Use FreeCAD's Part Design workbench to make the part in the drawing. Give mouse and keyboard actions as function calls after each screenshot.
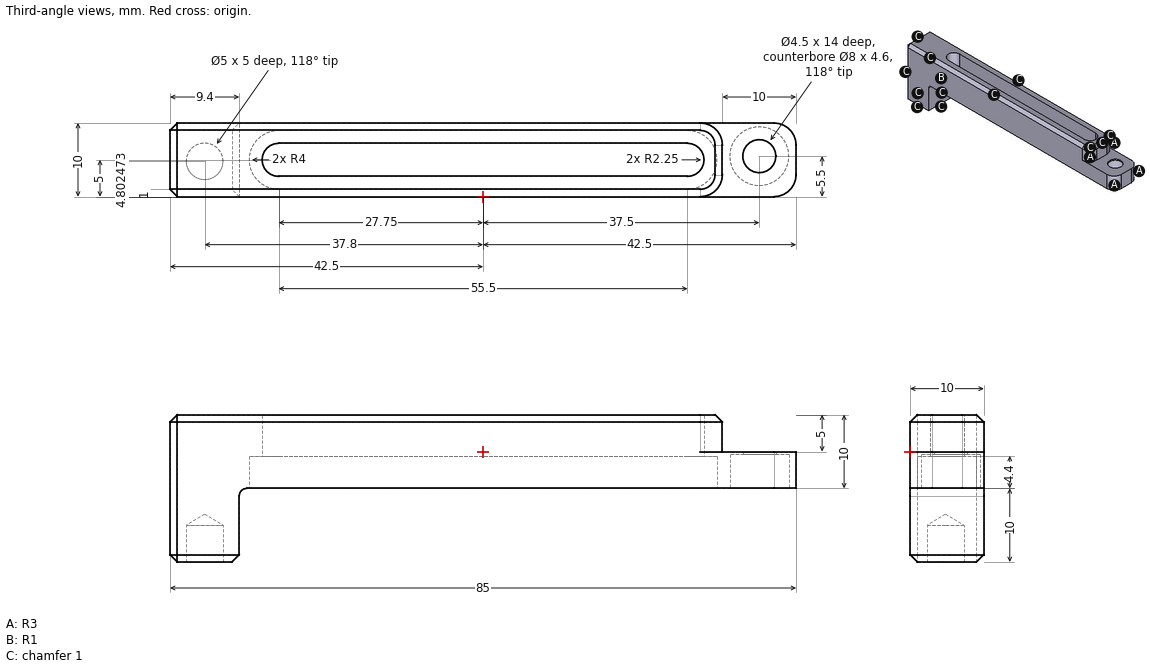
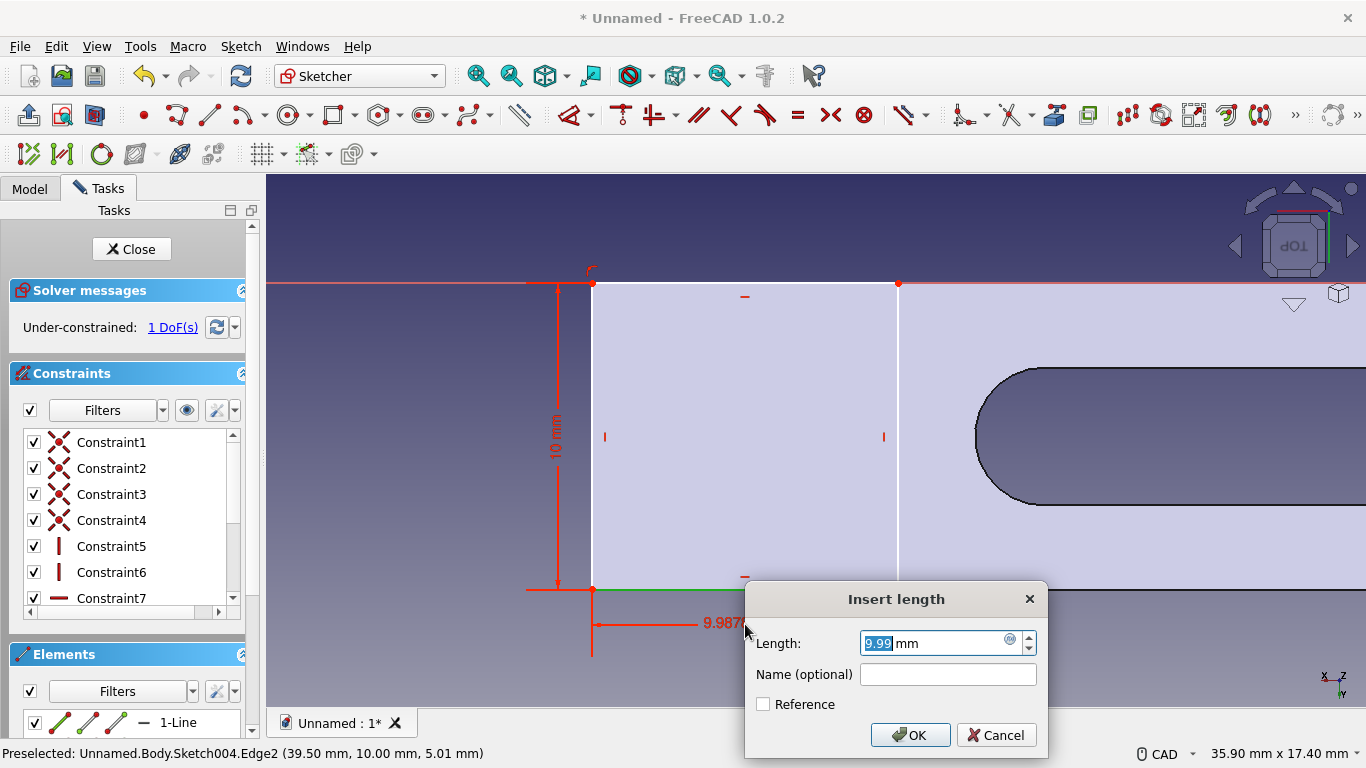
text(10)
key(Return)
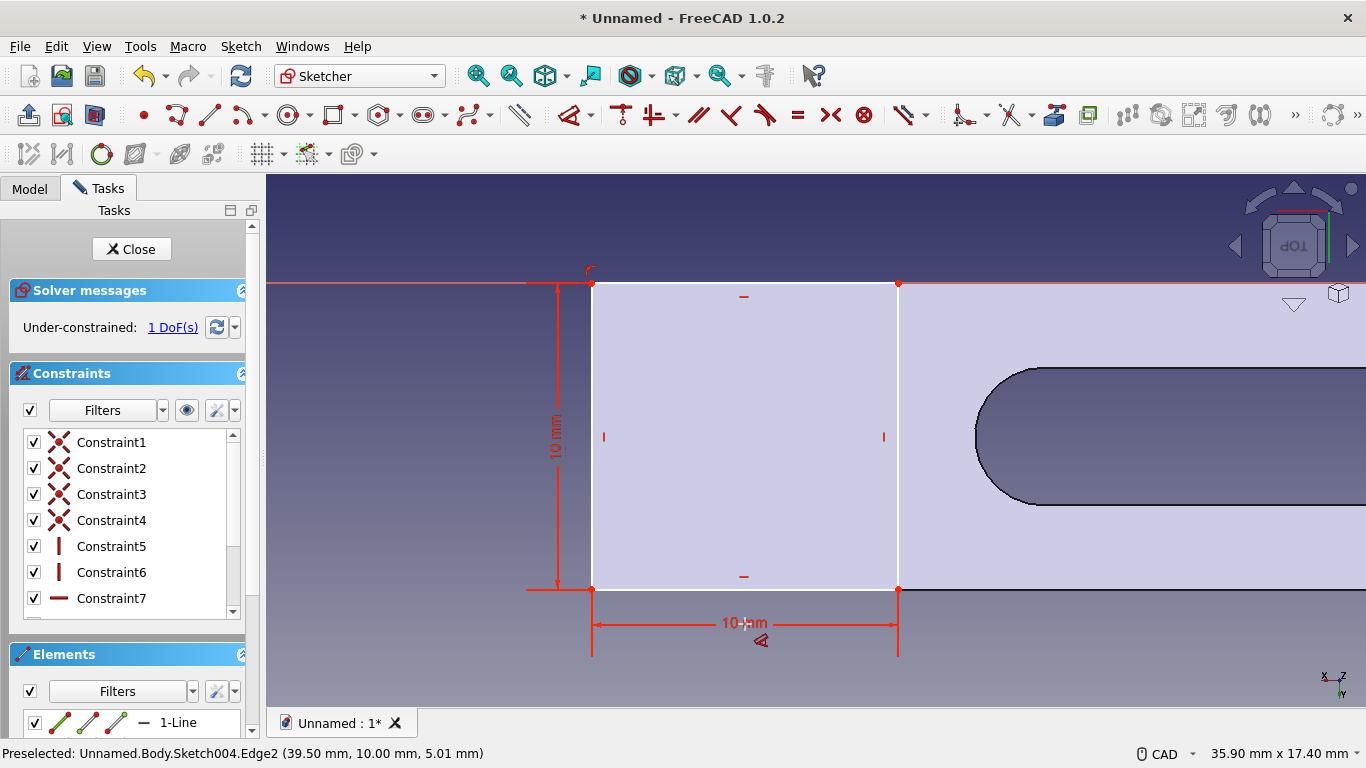
click(592, 283)
click(896, 249)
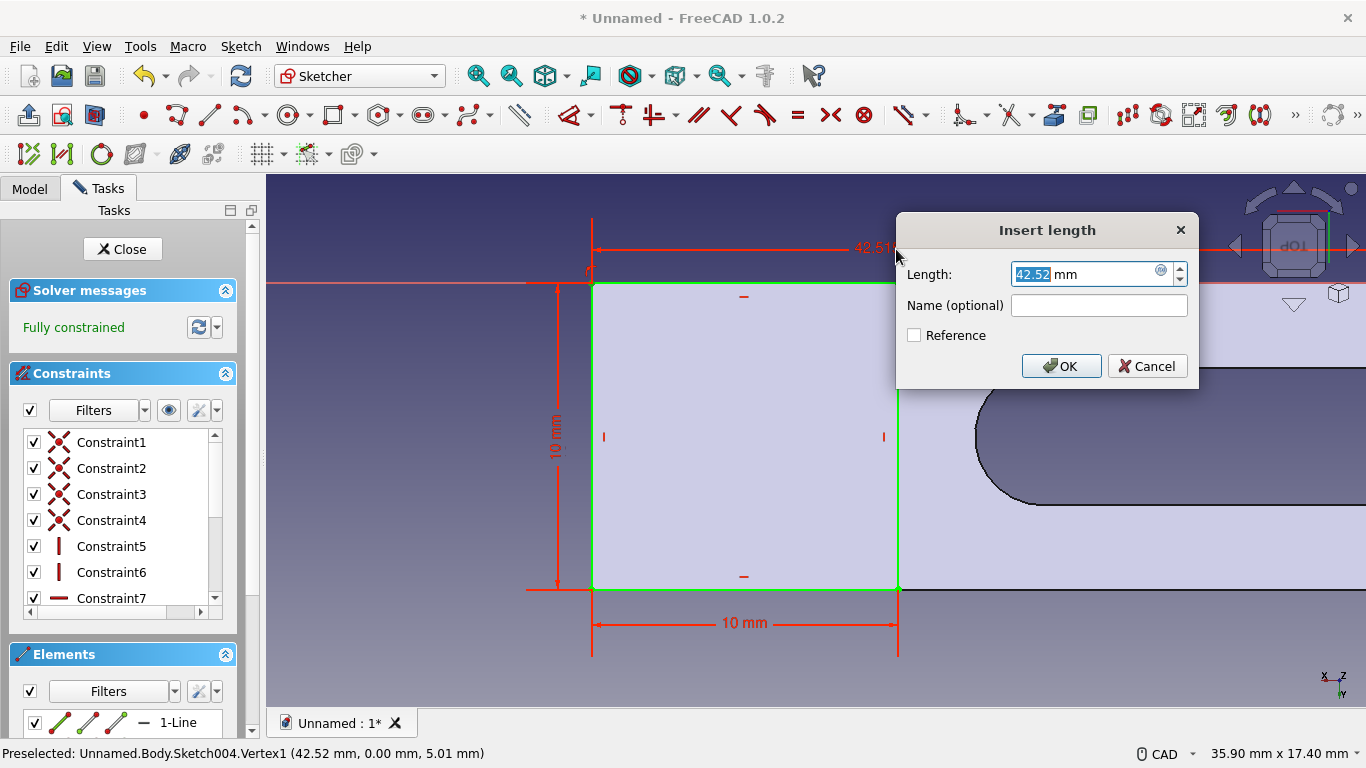
text(42.5)
key(Return)
key(Escape)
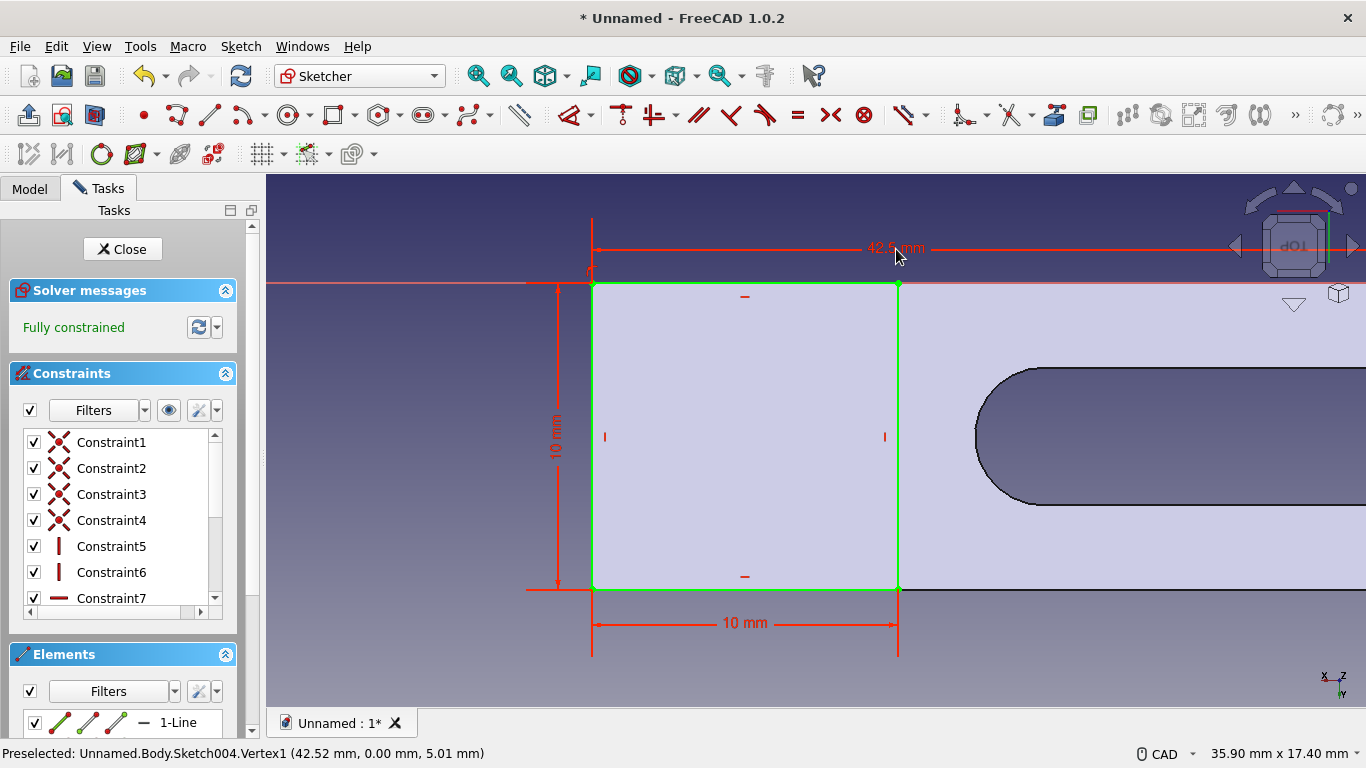
click(123, 249)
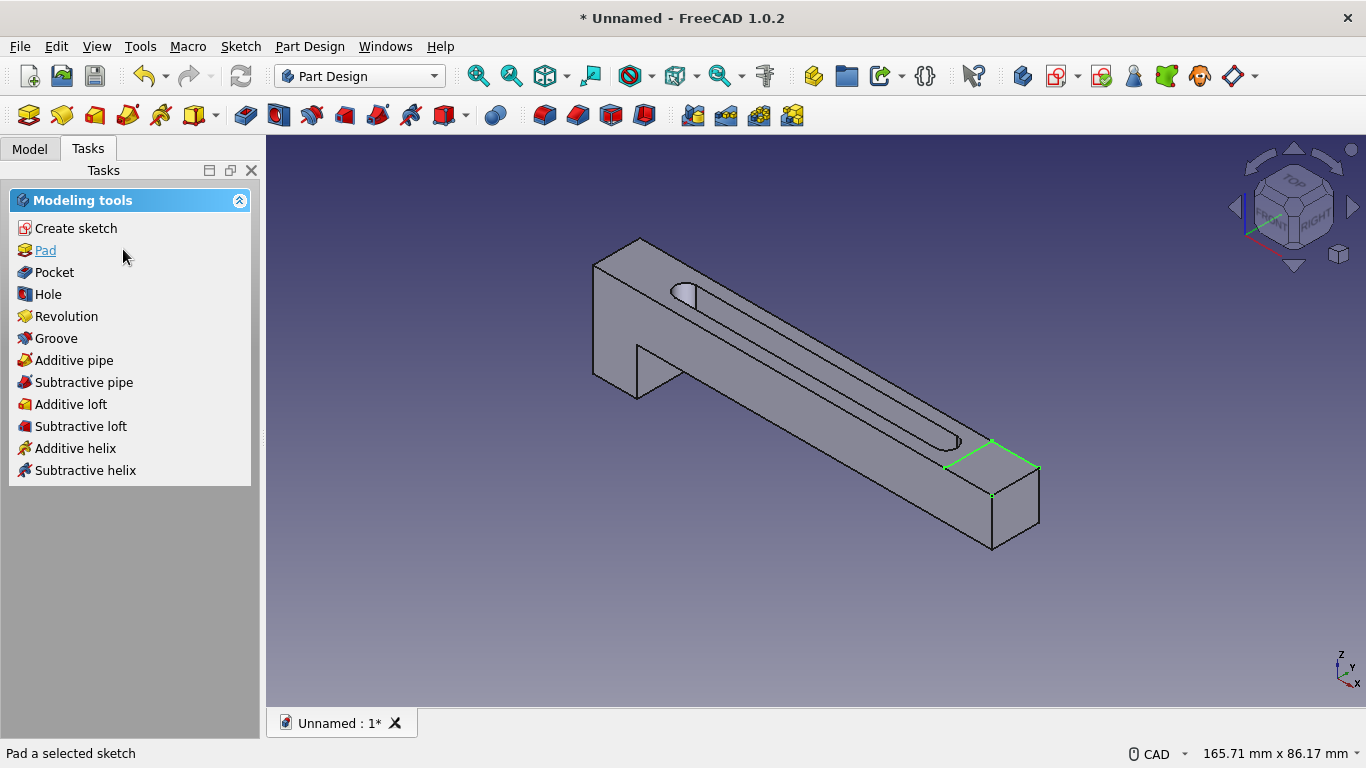
click(246, 116)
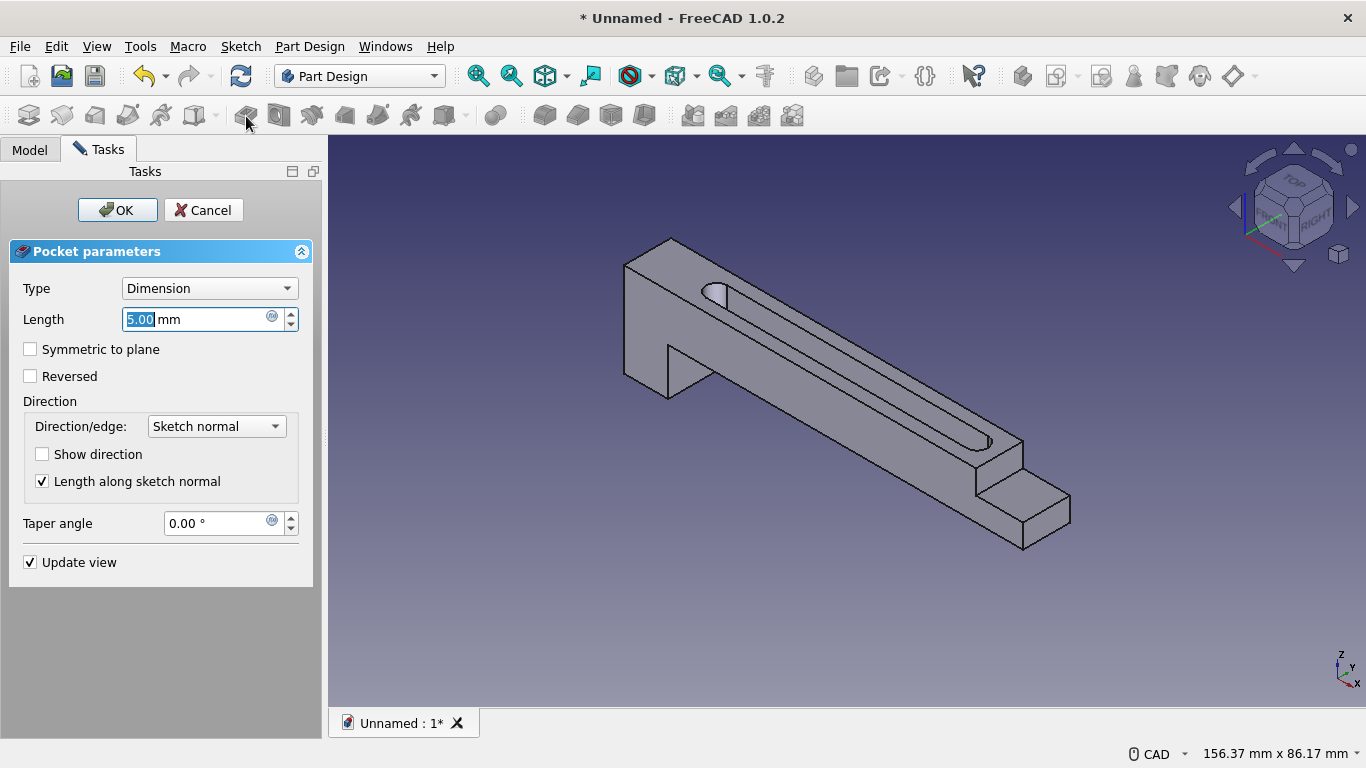
text(5)
key(Tab)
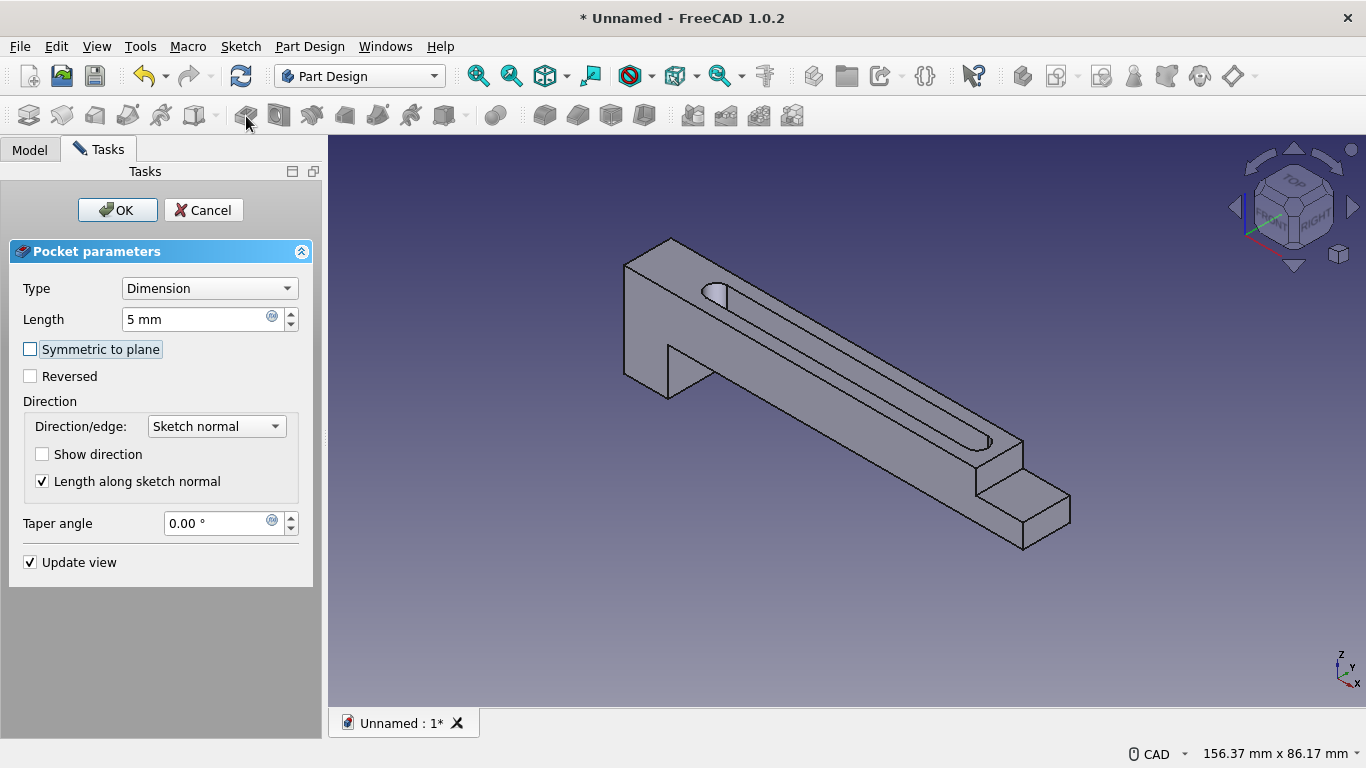
click(118, 210)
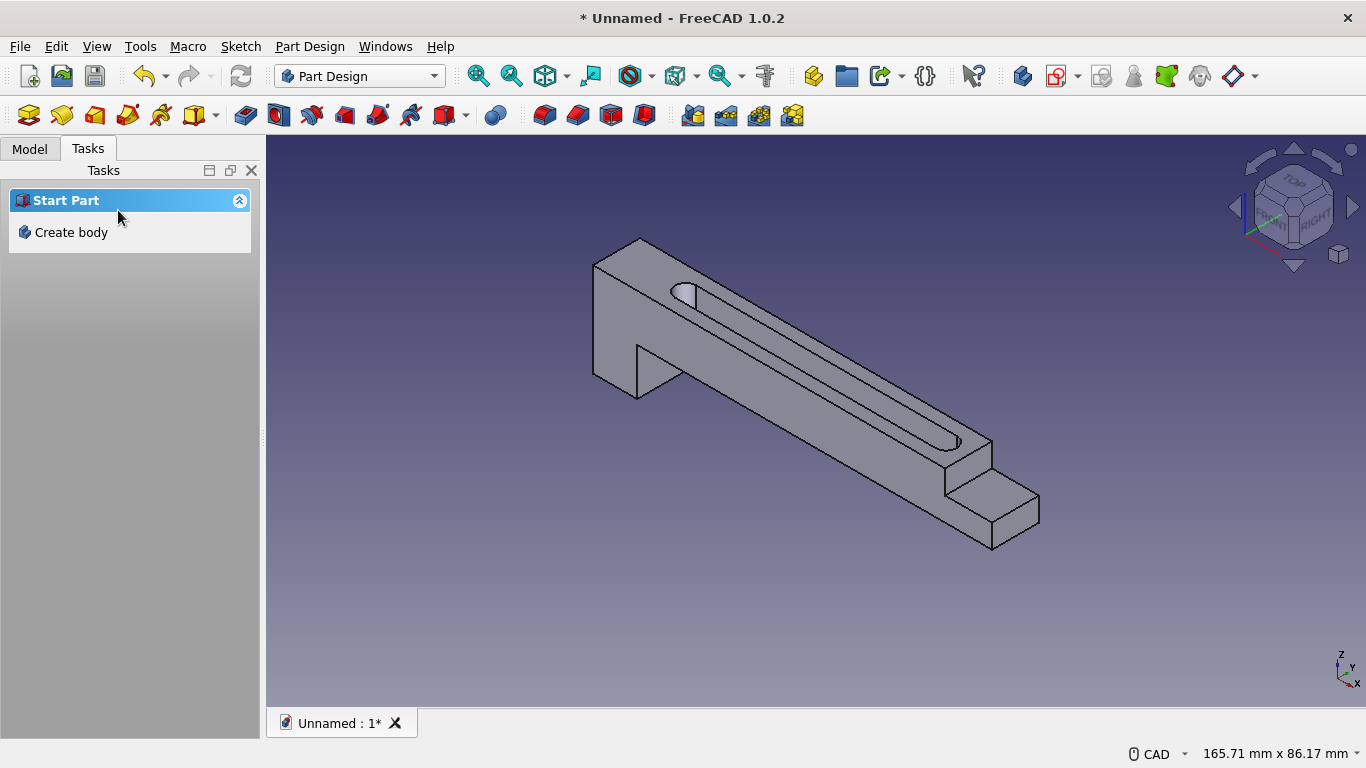
key(5)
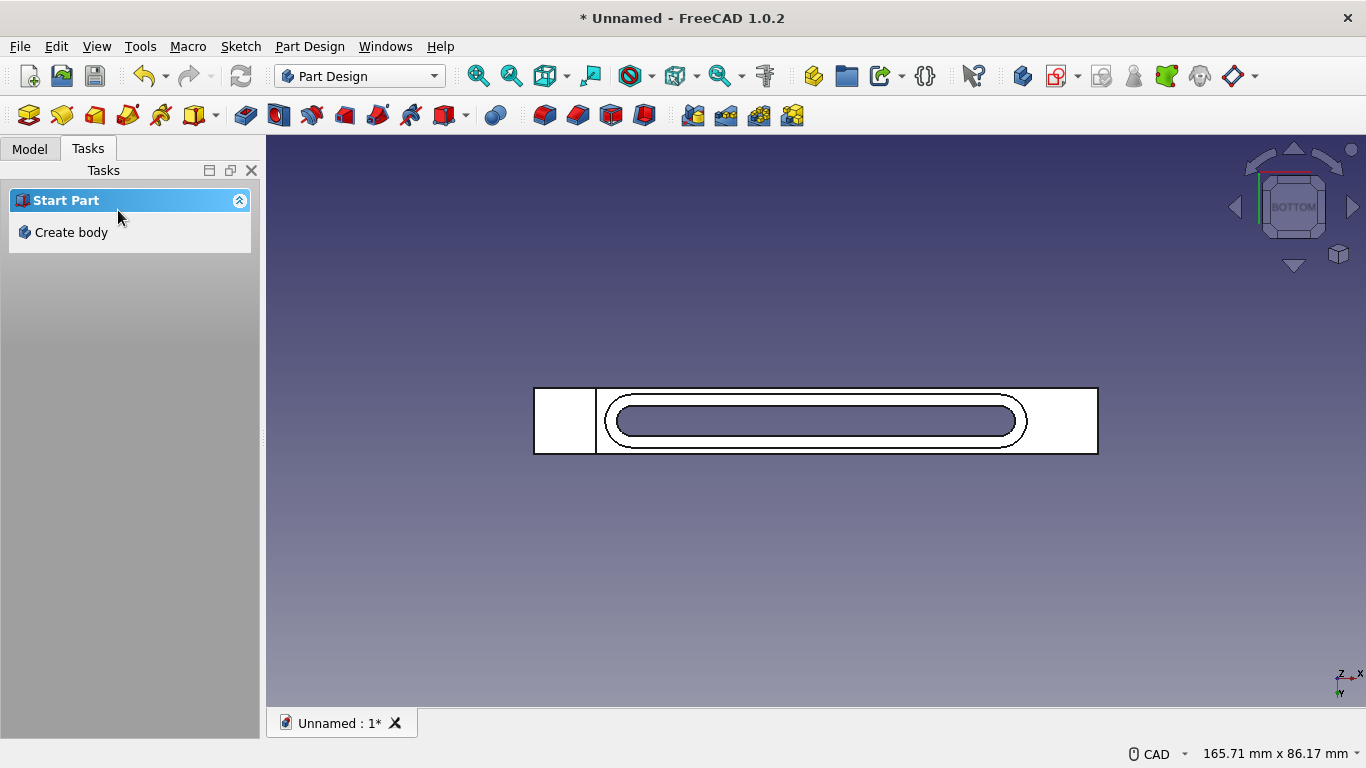
click(565, 420)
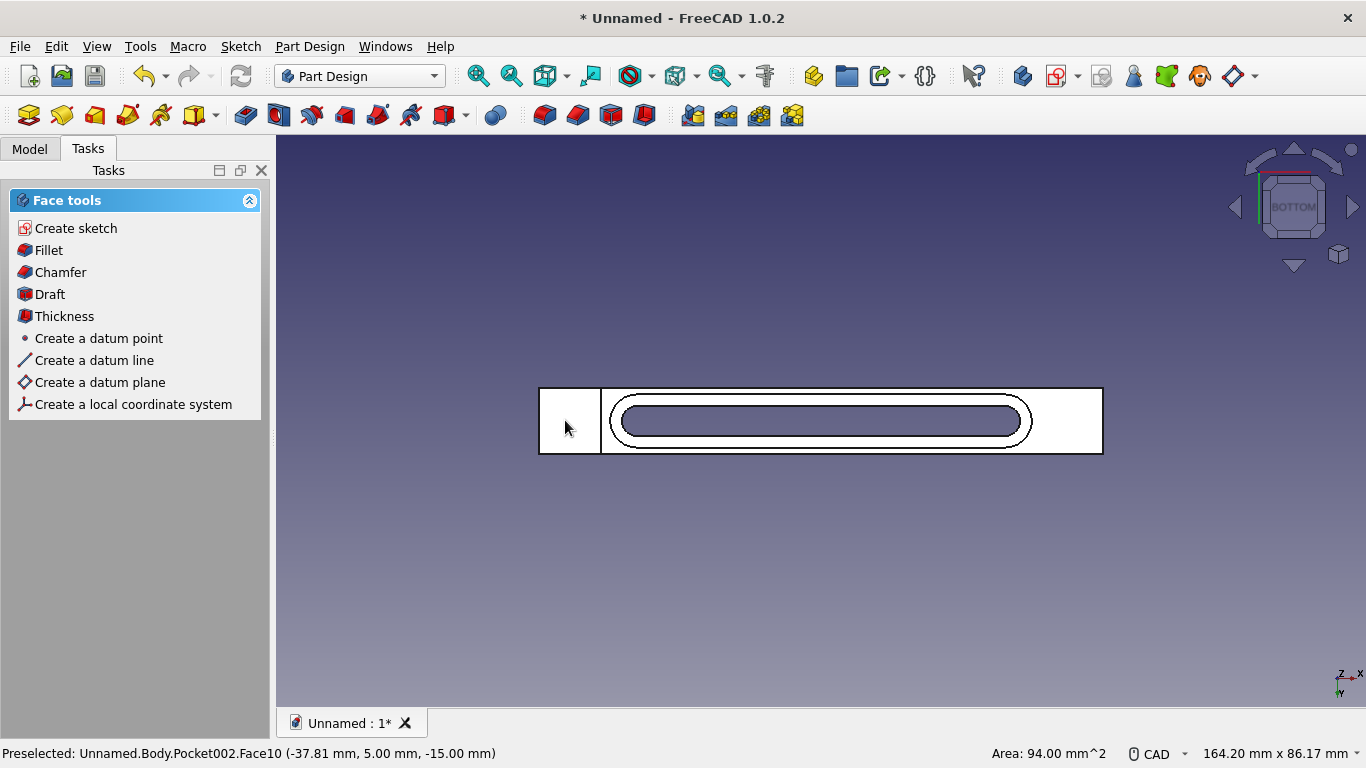
click(1056, 76)